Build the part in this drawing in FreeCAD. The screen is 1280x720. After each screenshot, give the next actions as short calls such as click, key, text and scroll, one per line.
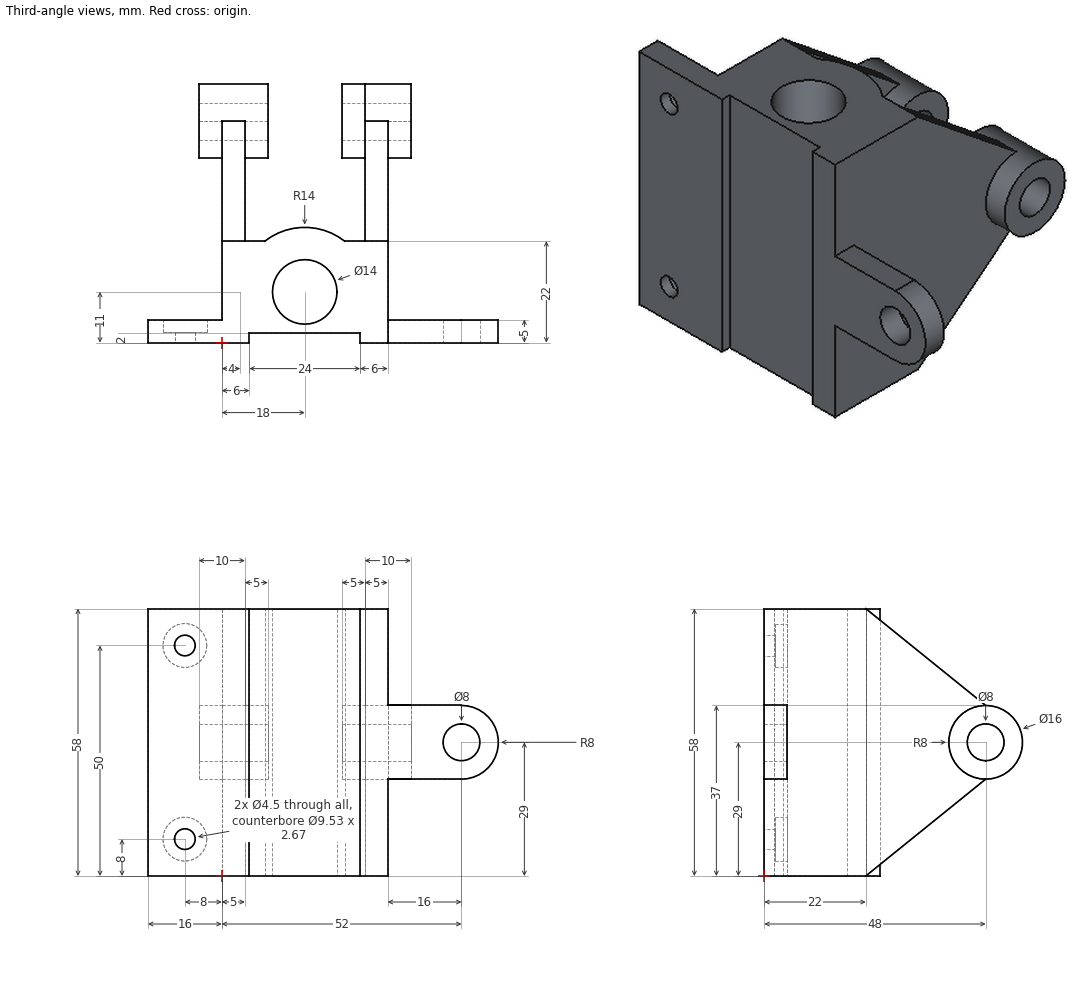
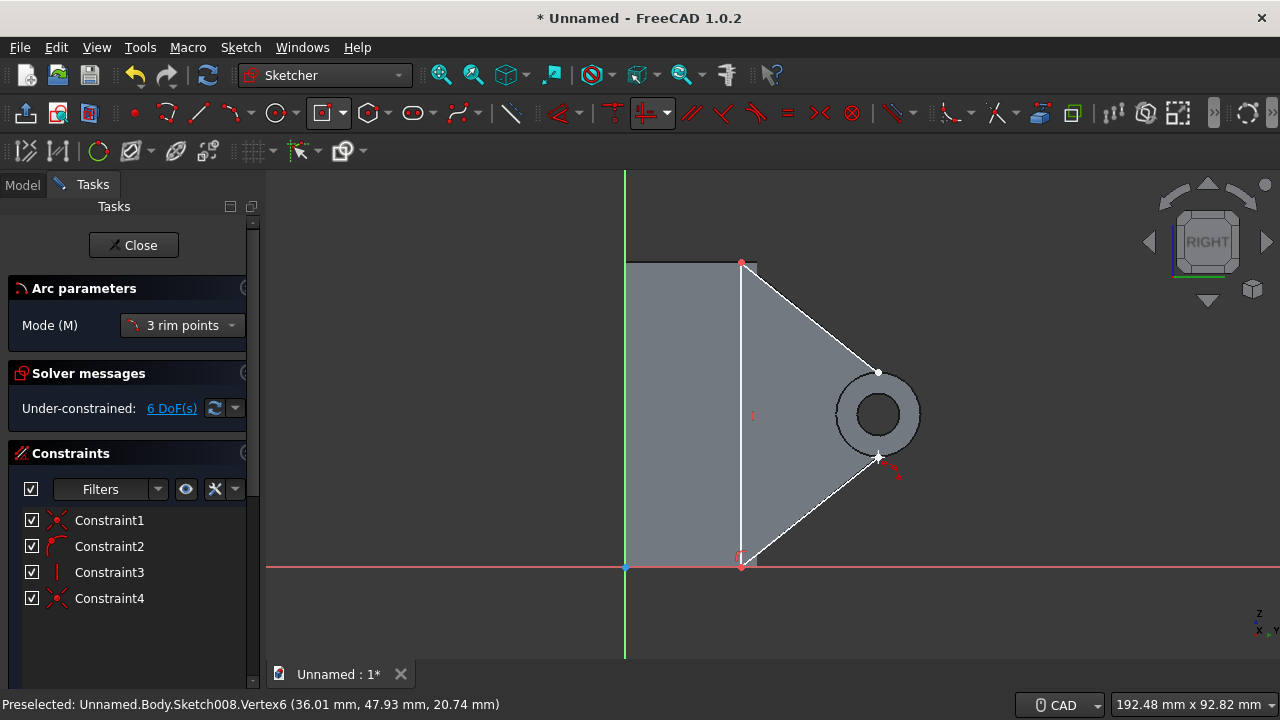
click(878, 458)
click(878, 373)
click(836, 414)
key(Escape)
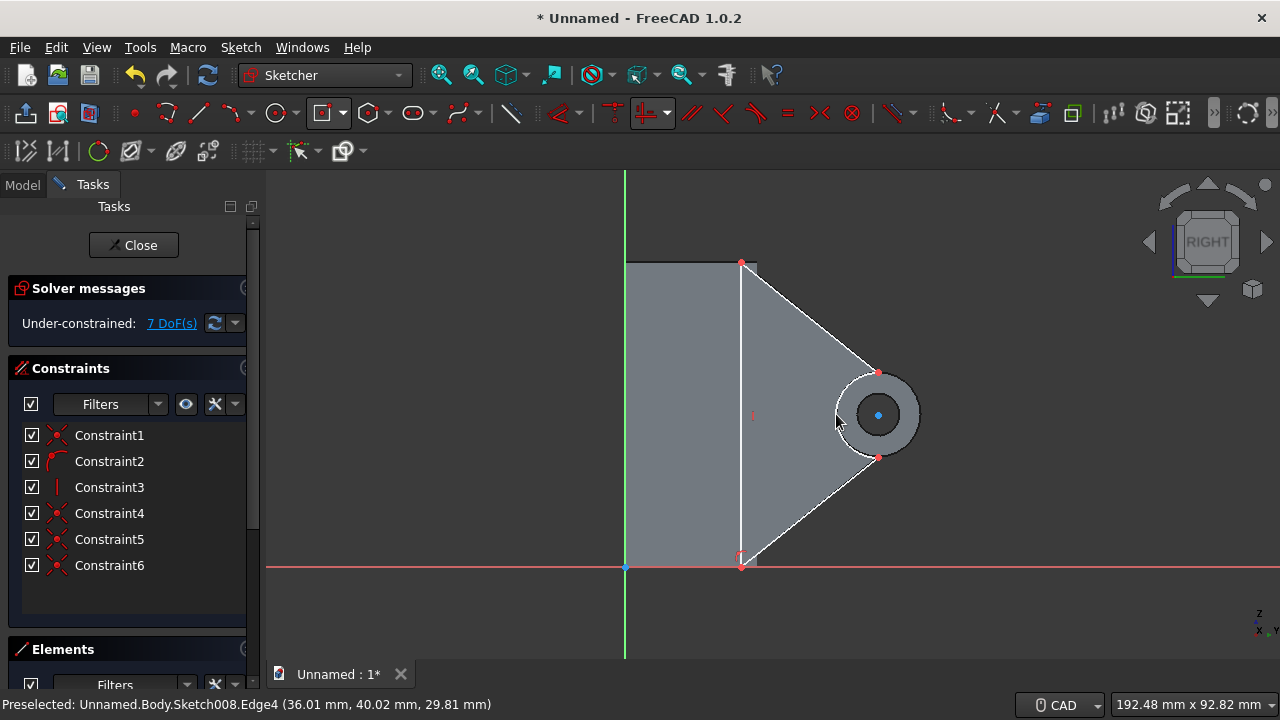
click(558, 114)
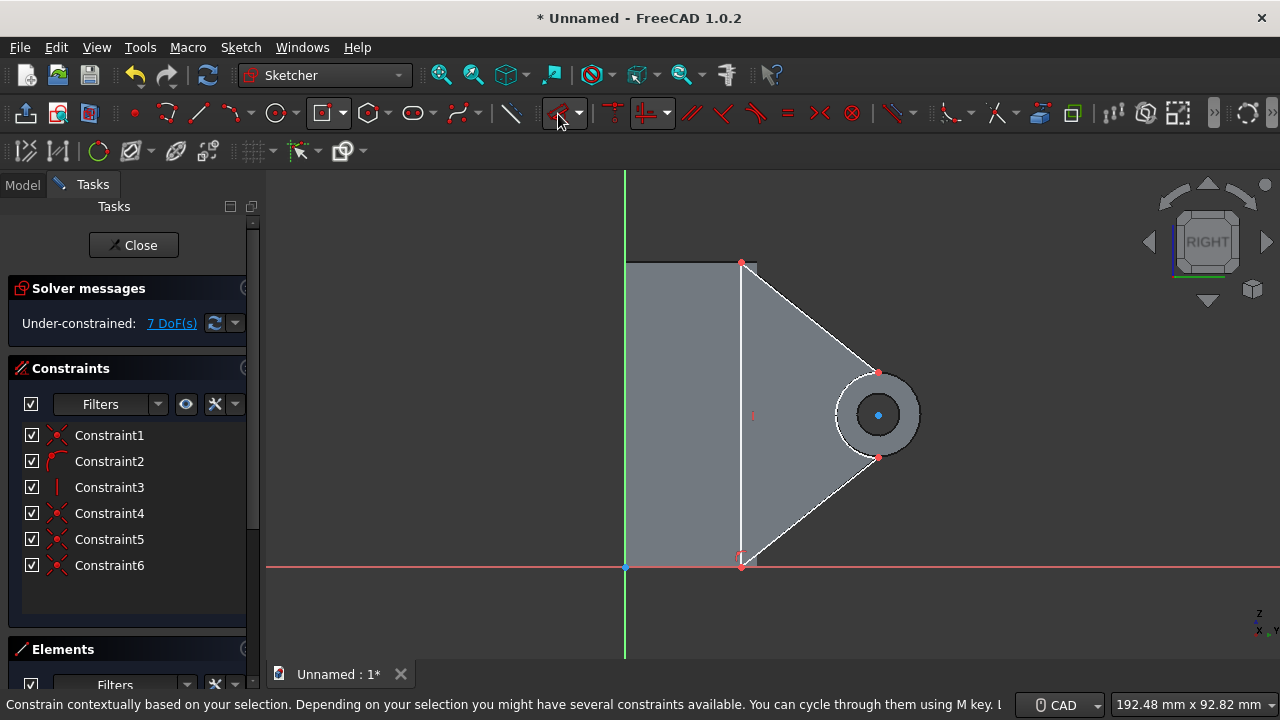
click(844, 391)
click(818, 372)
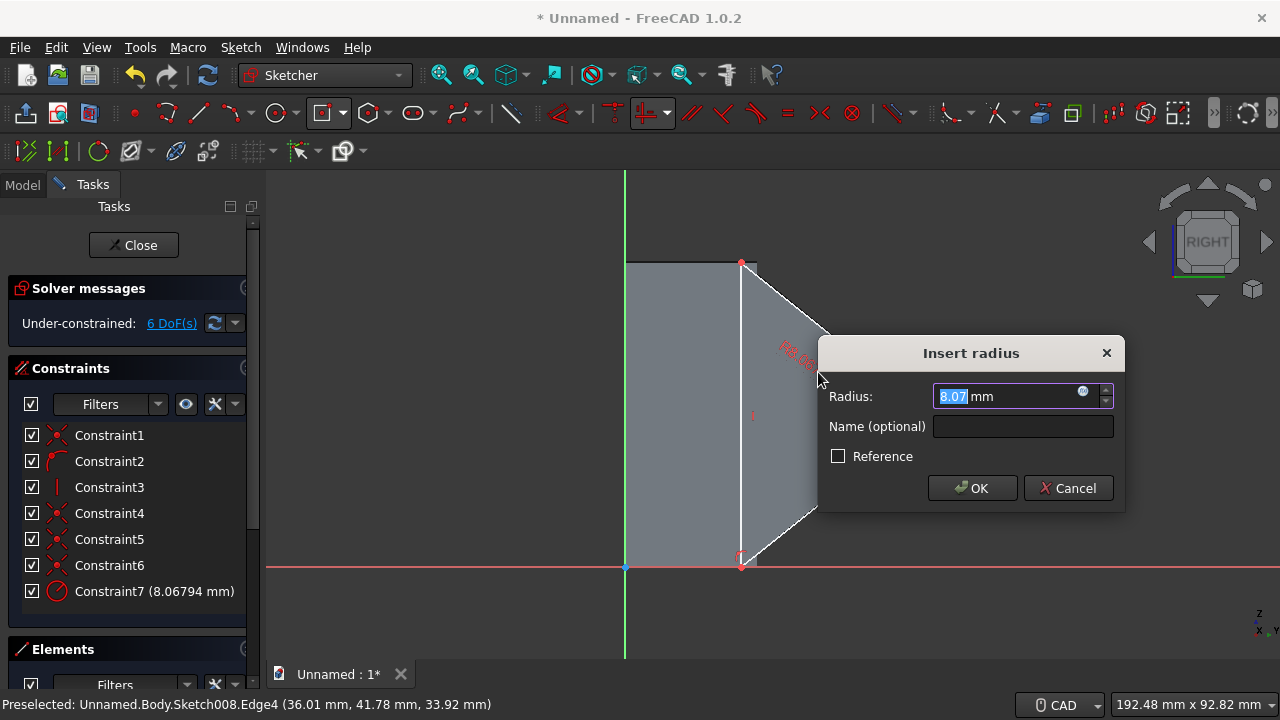
text(8)
key(Return)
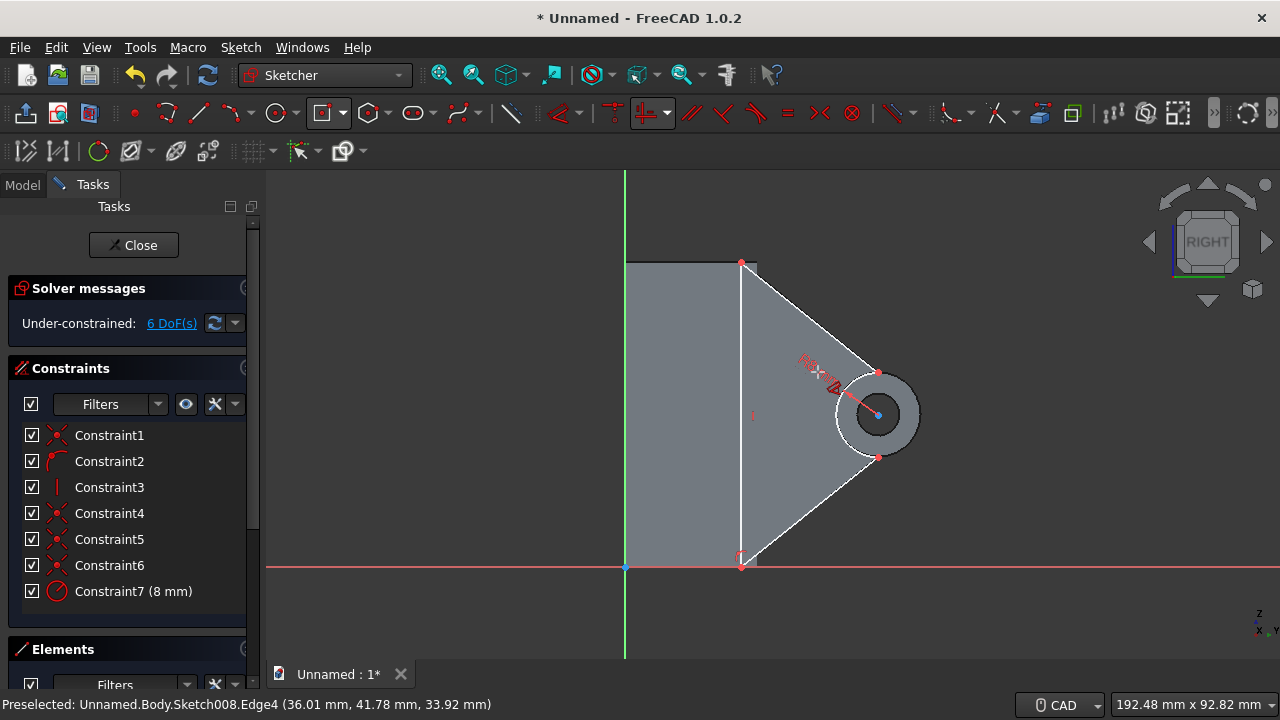
click(741, 354)
click(707, 415)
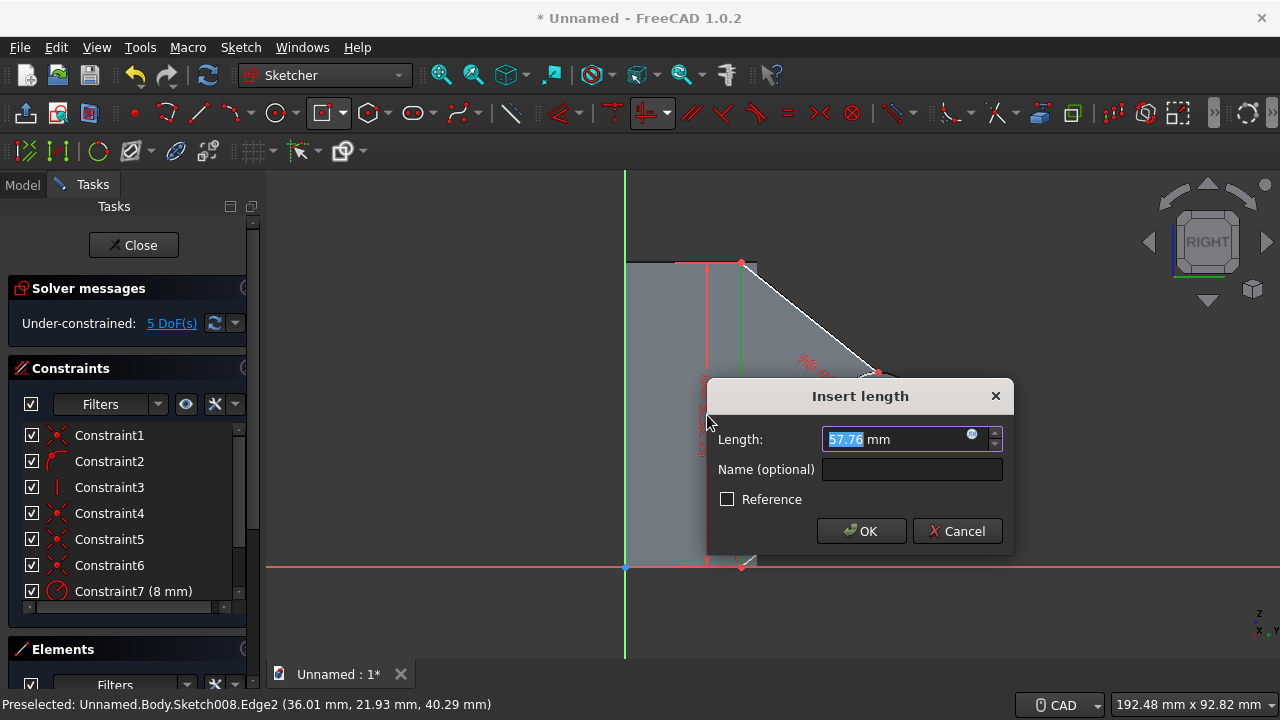
text(58)
key(Return)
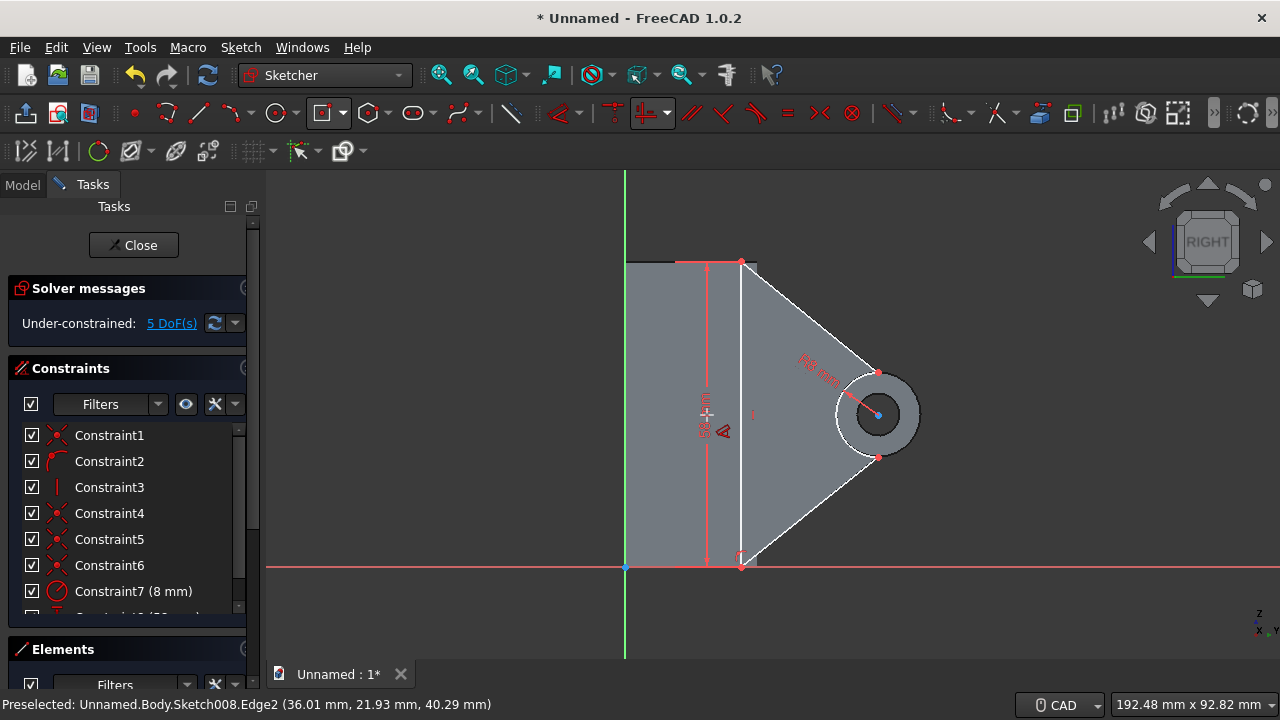
click(878, 373)
click(752, 601)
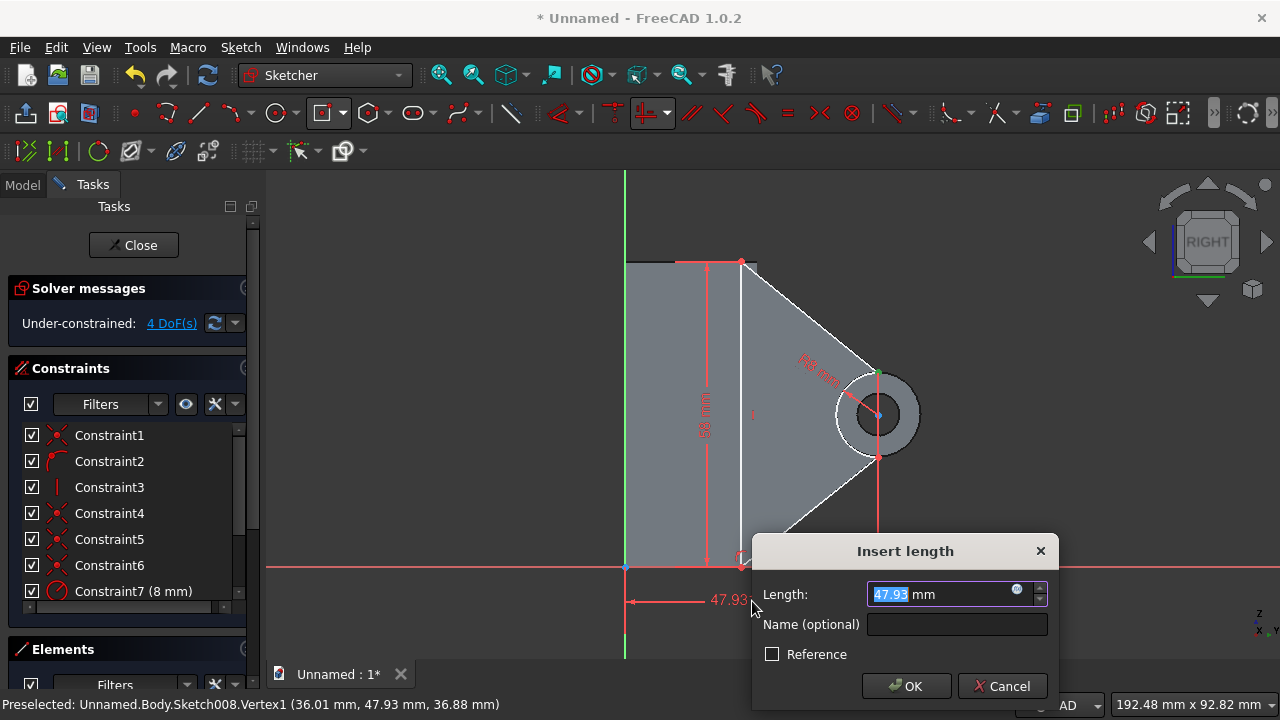
text(48)
key(Return)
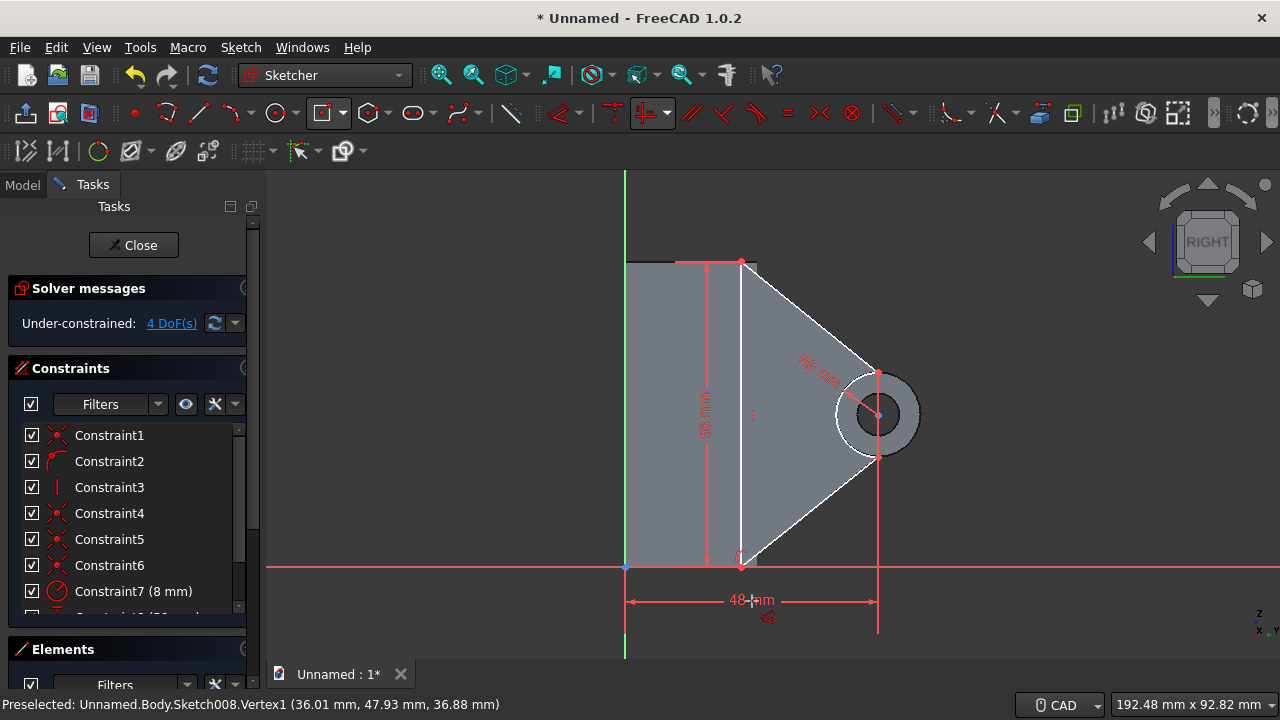
click(878, 373)
click(912, 470)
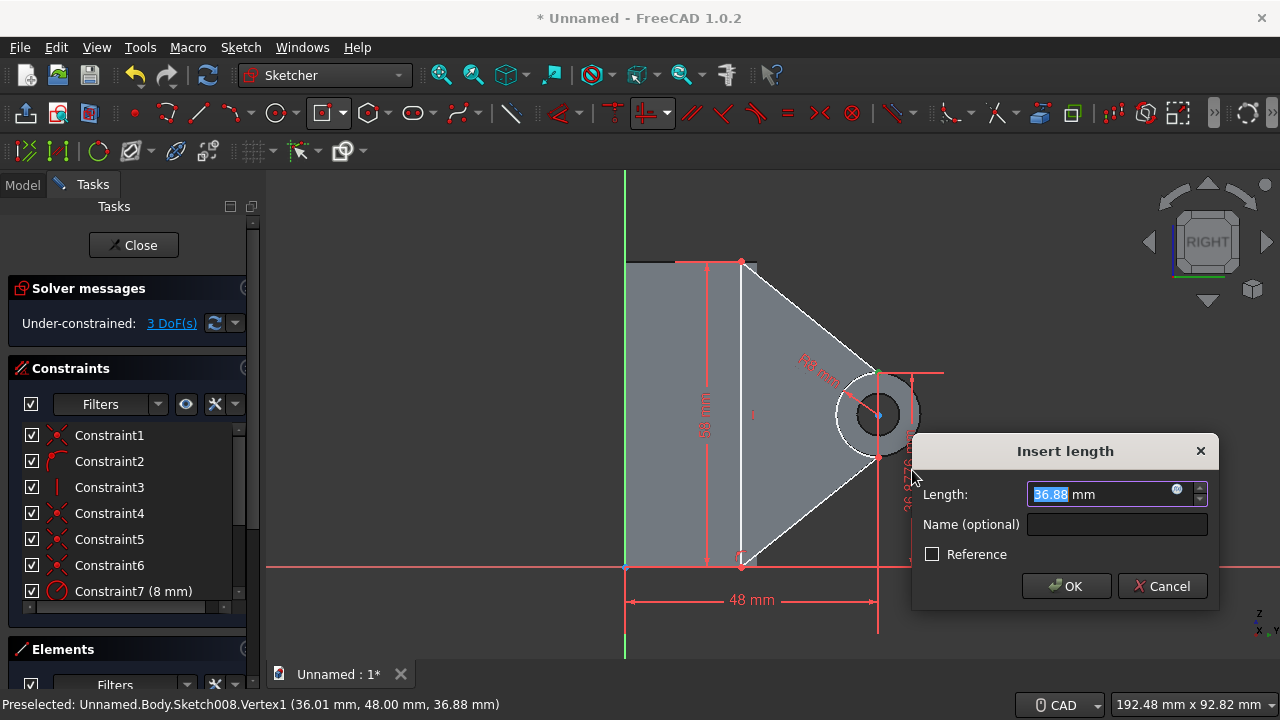
text(37)
key(Return)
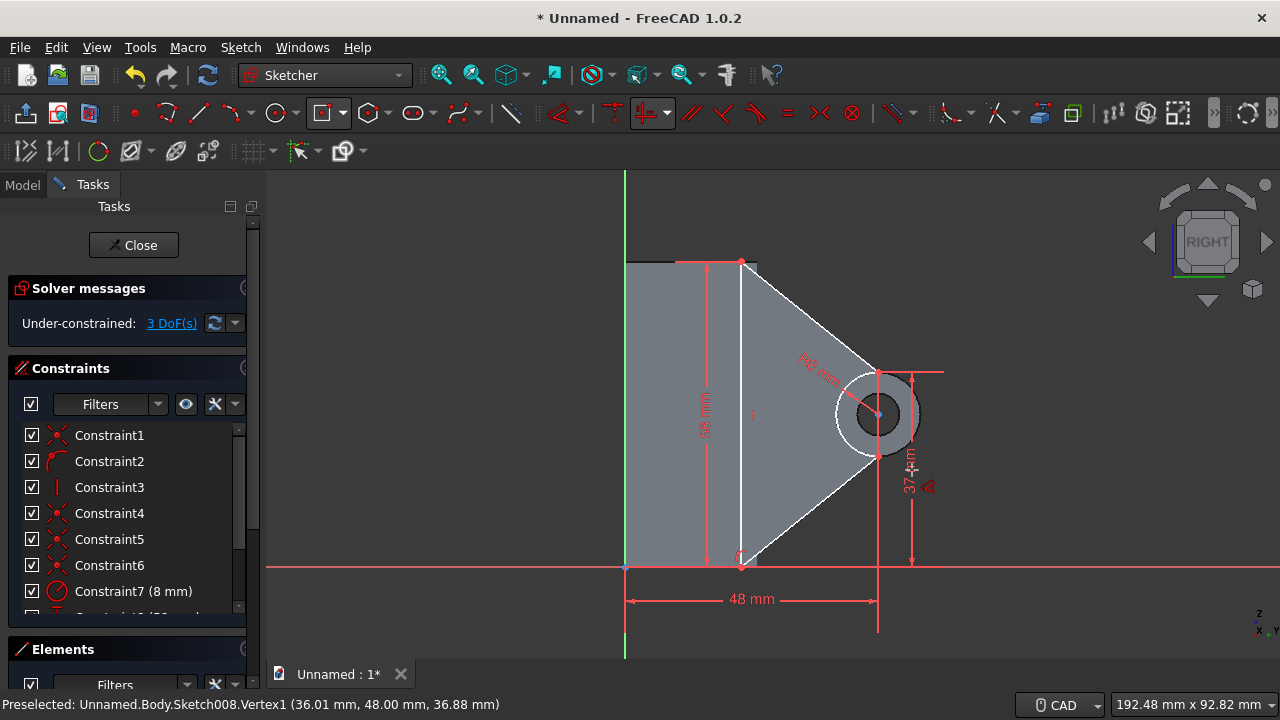
click(741, 262)
click(657, 601)